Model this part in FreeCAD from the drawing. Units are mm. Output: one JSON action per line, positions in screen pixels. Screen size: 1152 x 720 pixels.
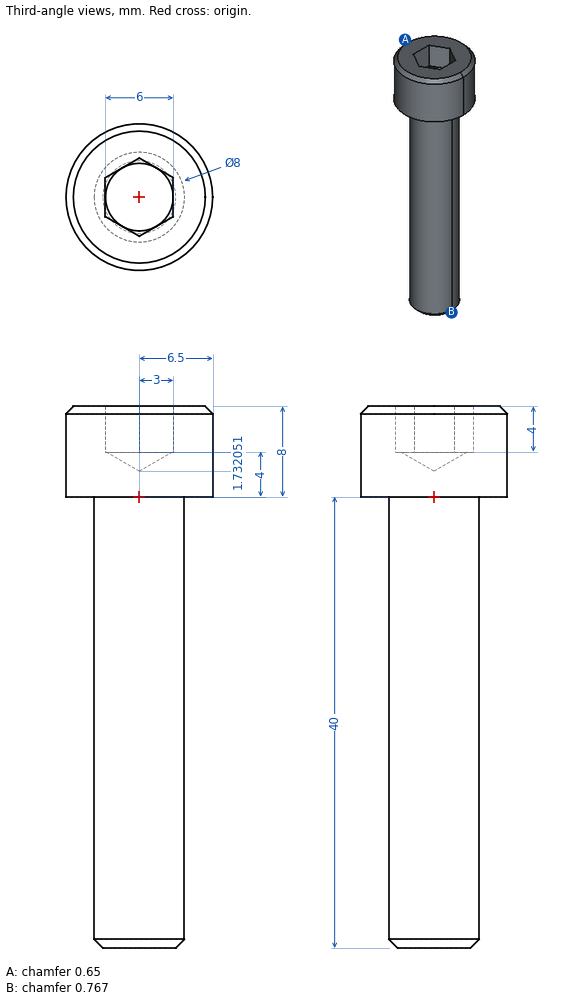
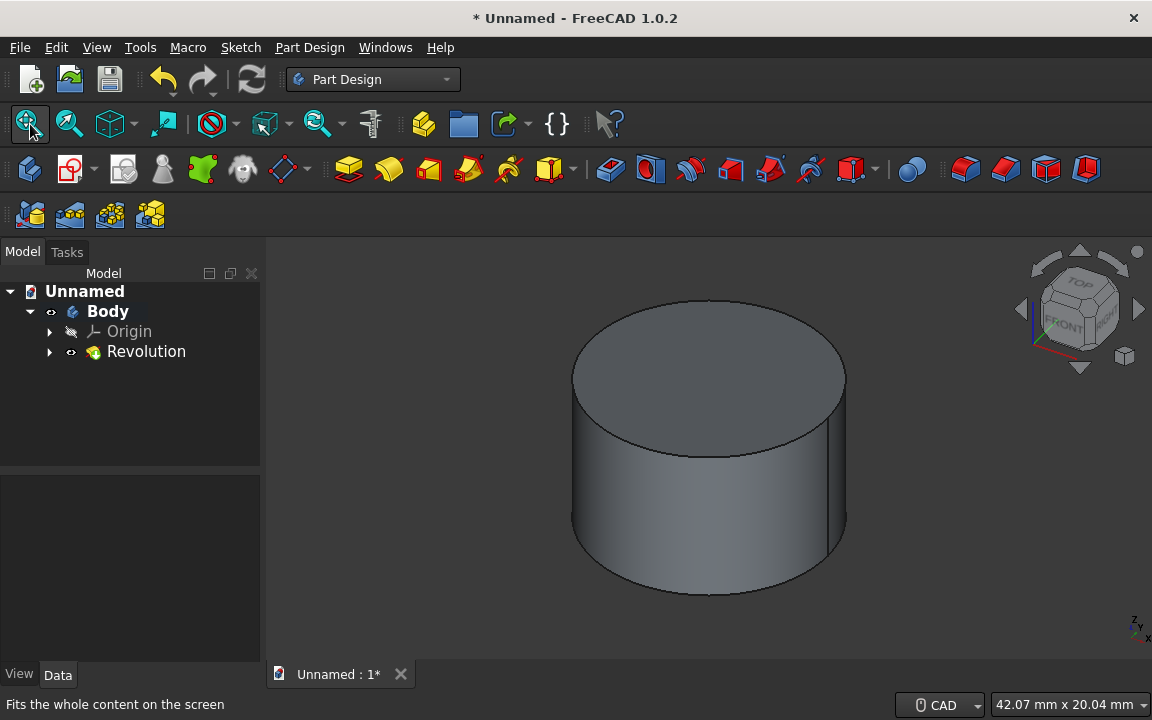
{"action": "key", "text": "5"}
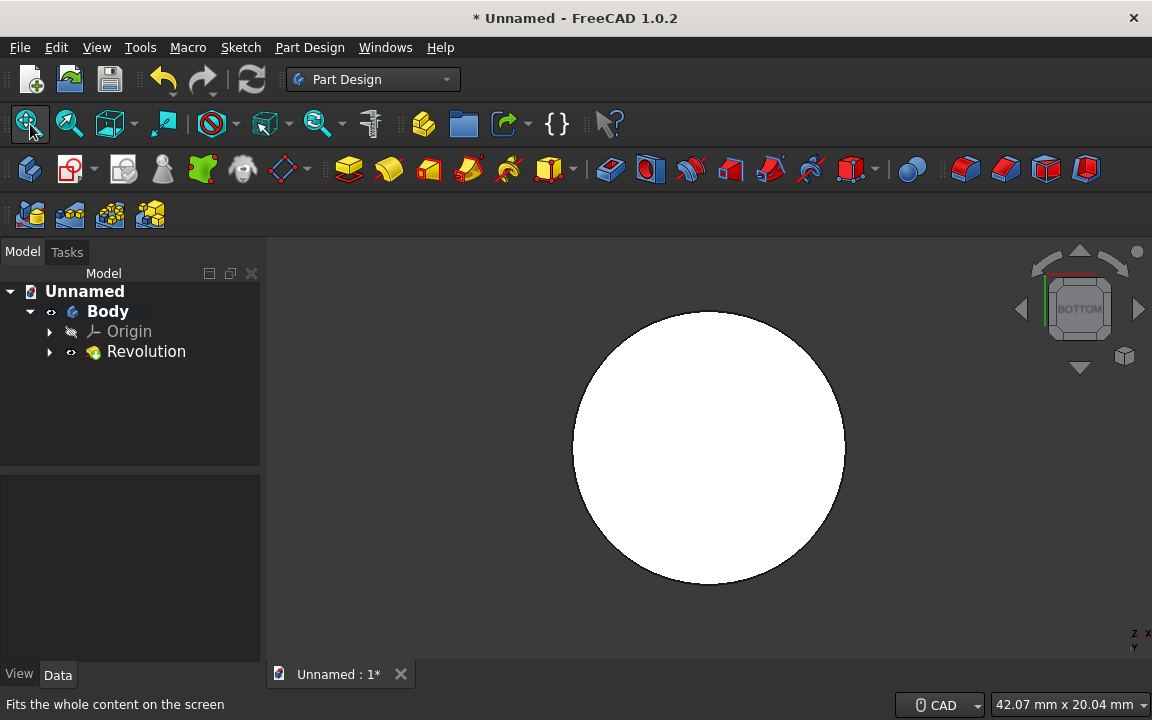
{"action": "left_click", "coordinate": [709, 447]}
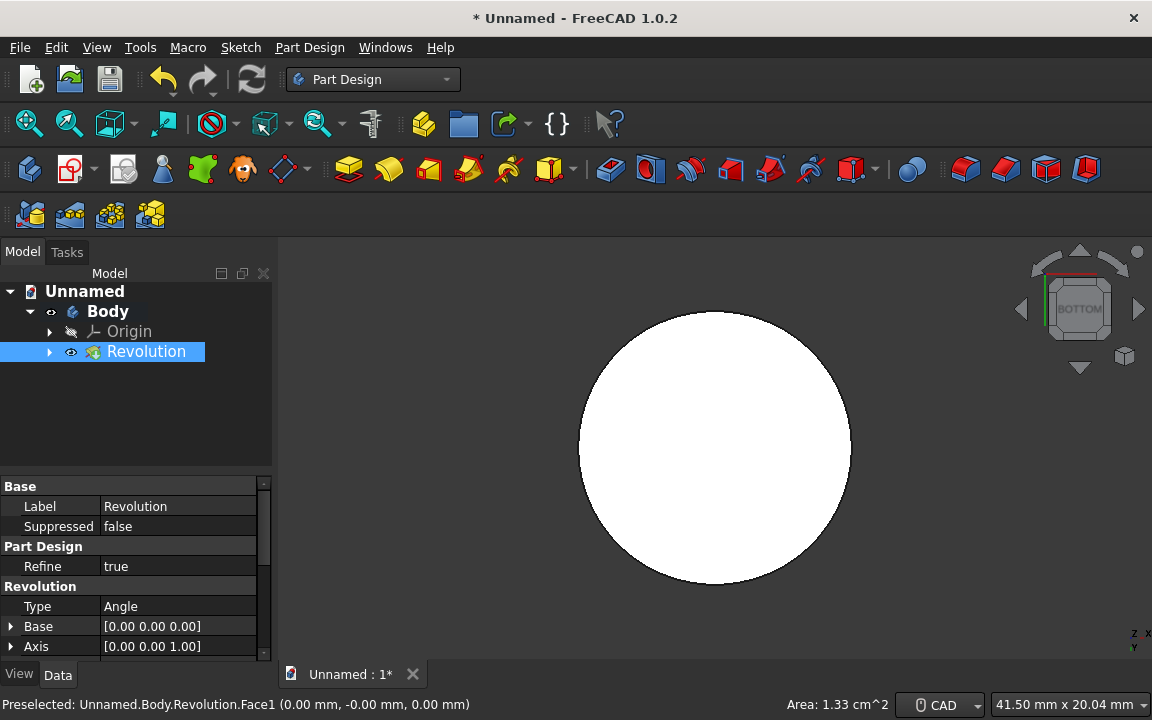
{"action": "left_click", "coordinate": [70, 170]}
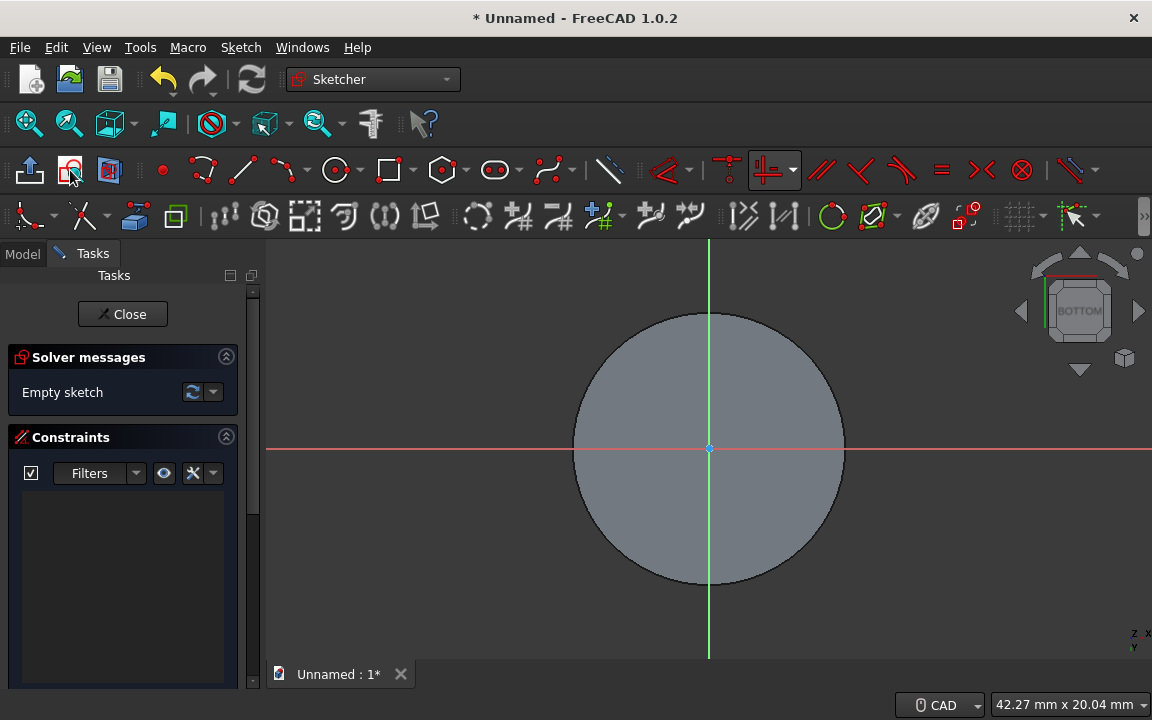
{"action": "scroll", "coordinate": [848, 449], "scroll_direction": "up", "scroll_amount": 2}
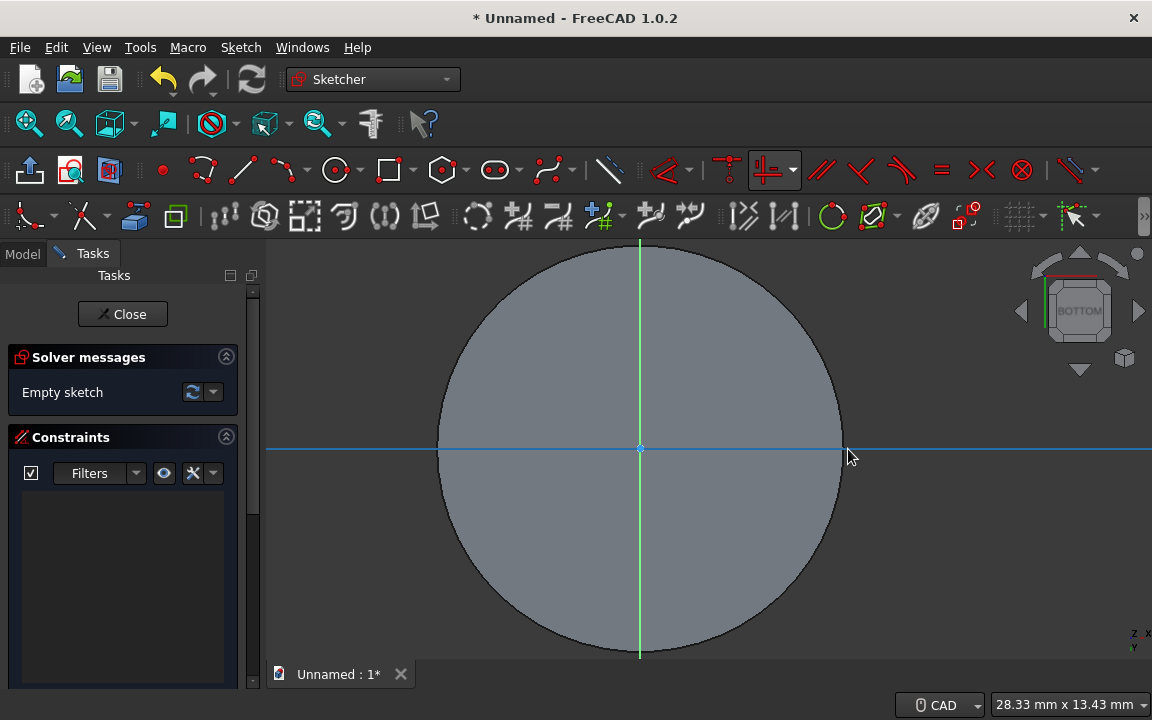
{"action": "left_click", "coordinate": [336, 170]}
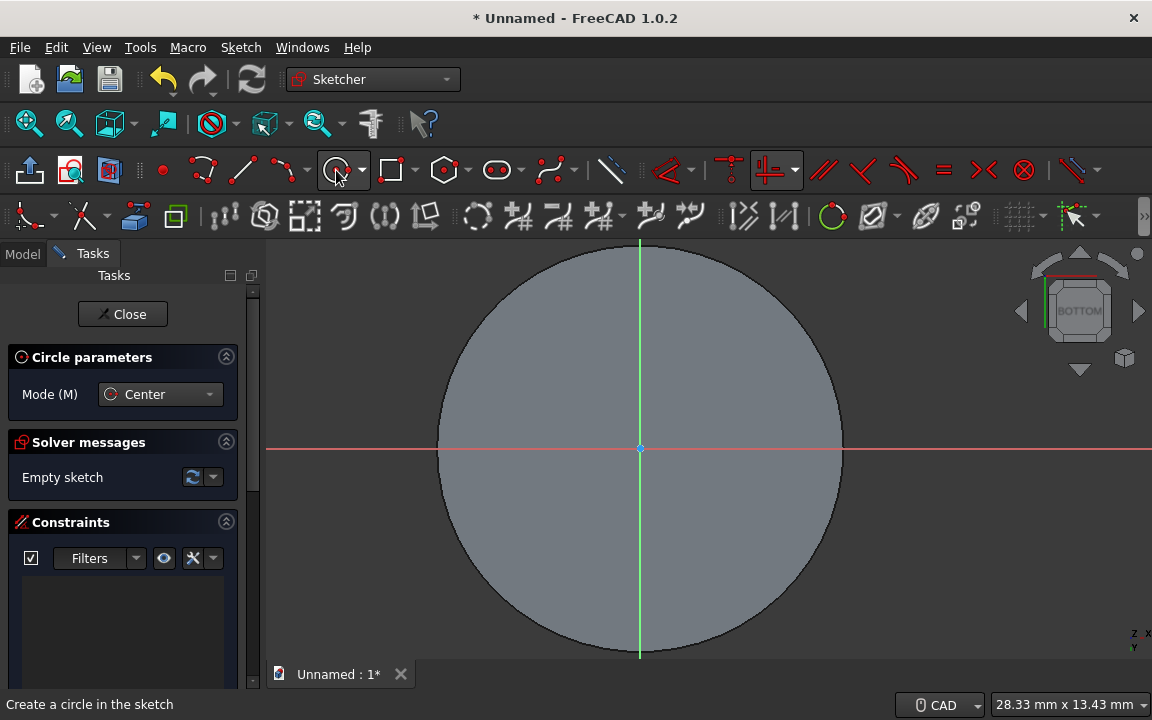
{"action": "left_click", "coordinate": [640, 449]}
{"action": "mouse_move", "coordinate": [729, 360]}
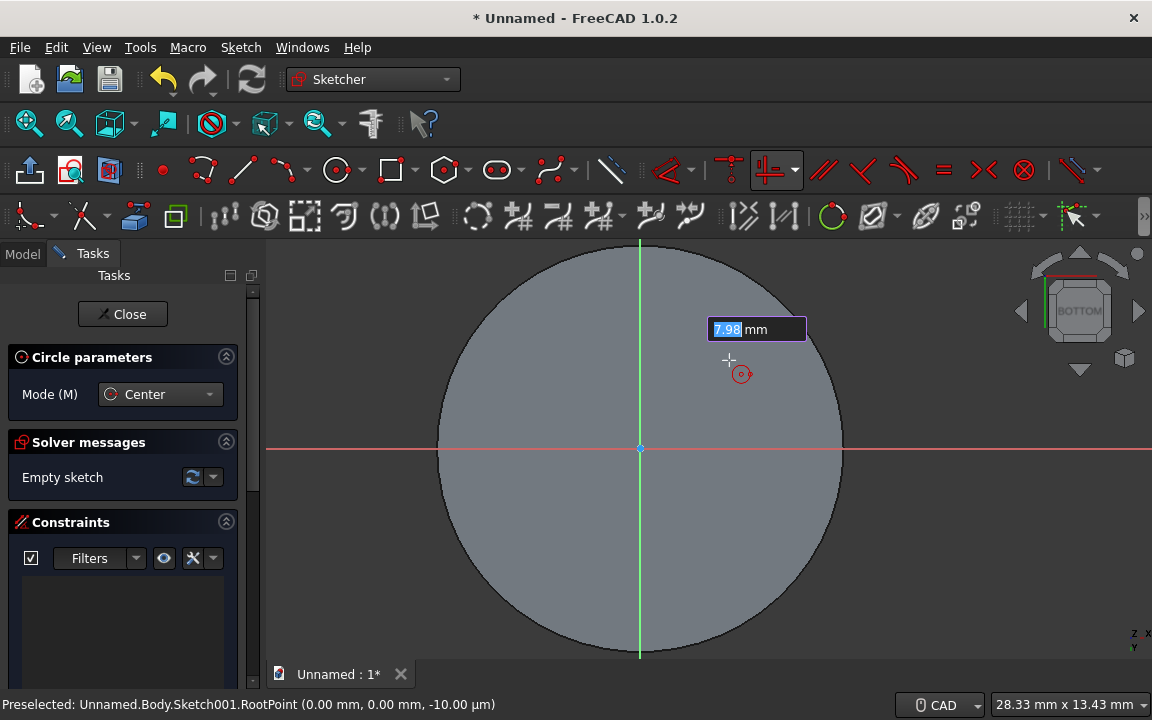
{"action": "type", "text": "8"}
{"action": "key", "text": "Return"}
{"action": "key", "text": "Escape"}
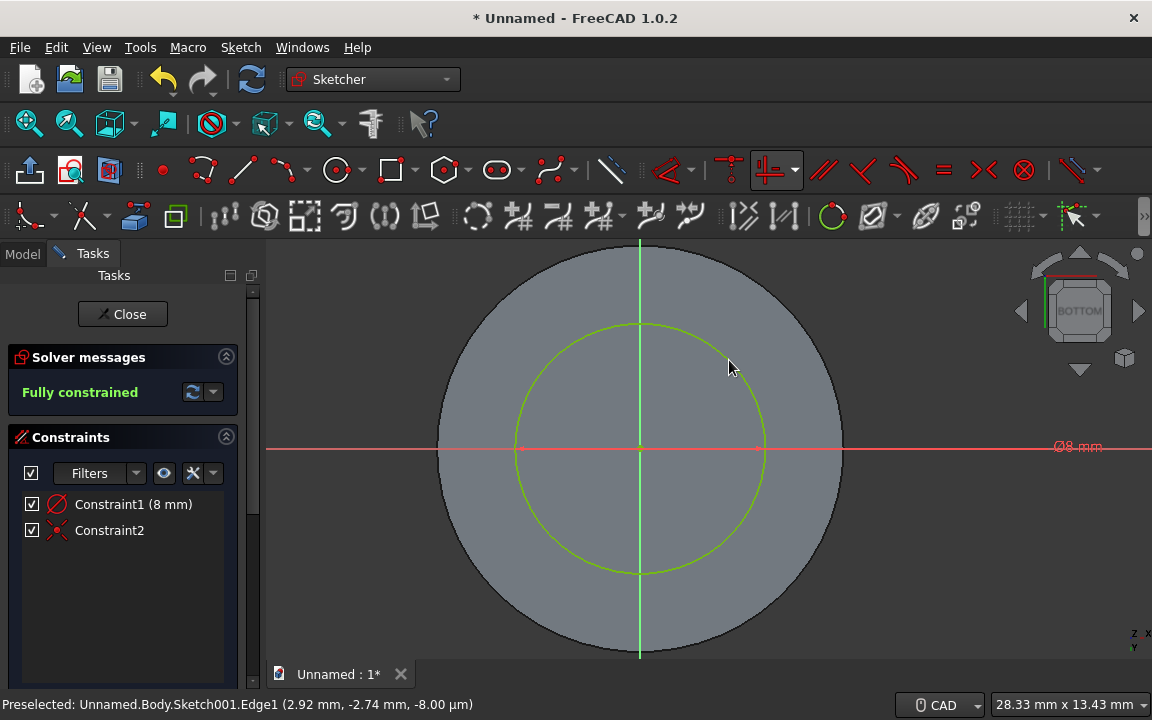
{"action": "left_click", "coordinate": [123, 314]}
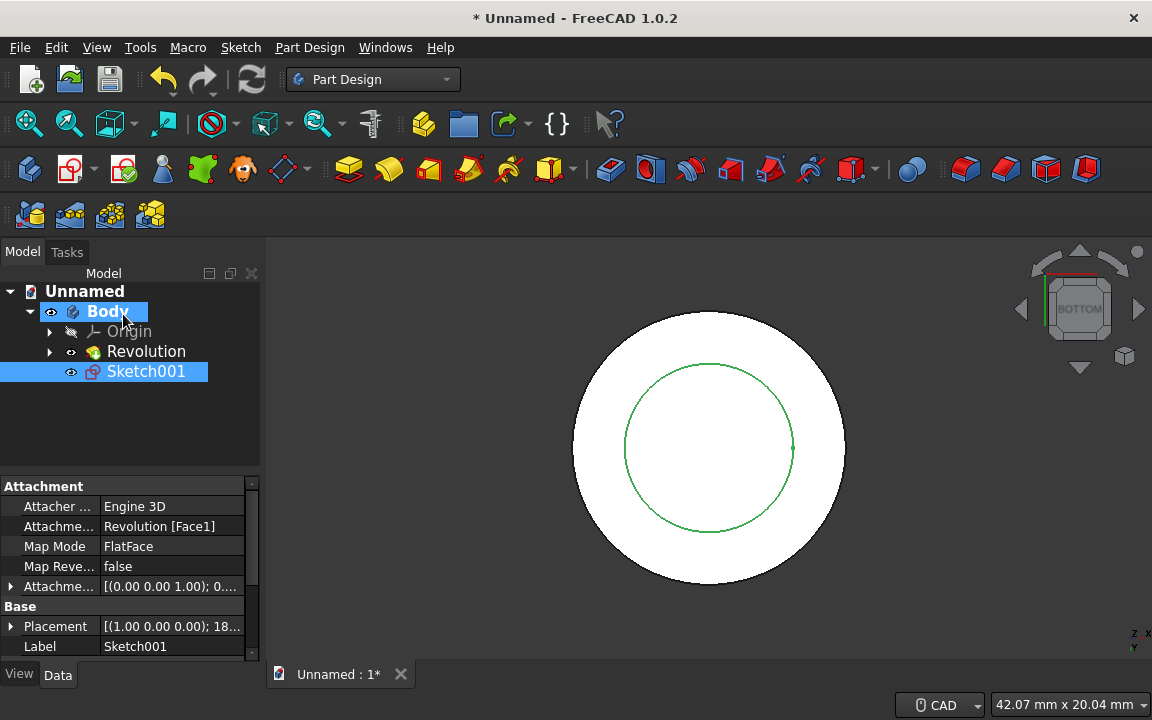
{"action": "left_click", "coordinate": [350, 170]}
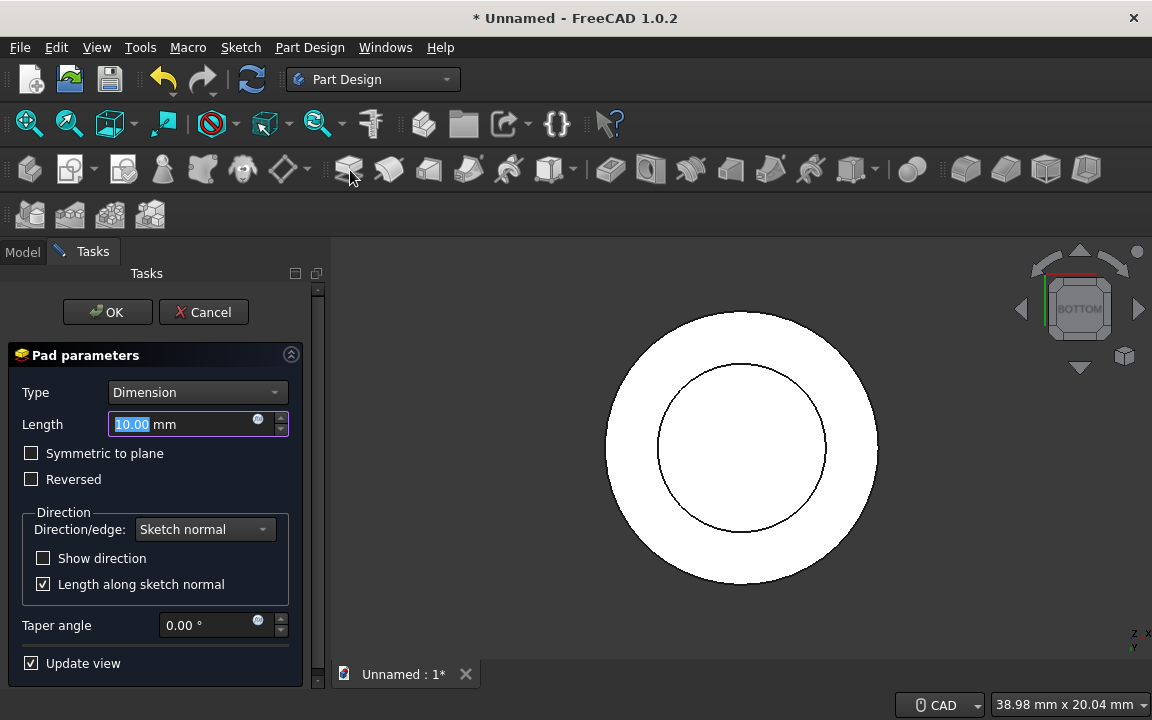
{"action": "type", "text": "40"}
{"action": "key", "text": "Tab"}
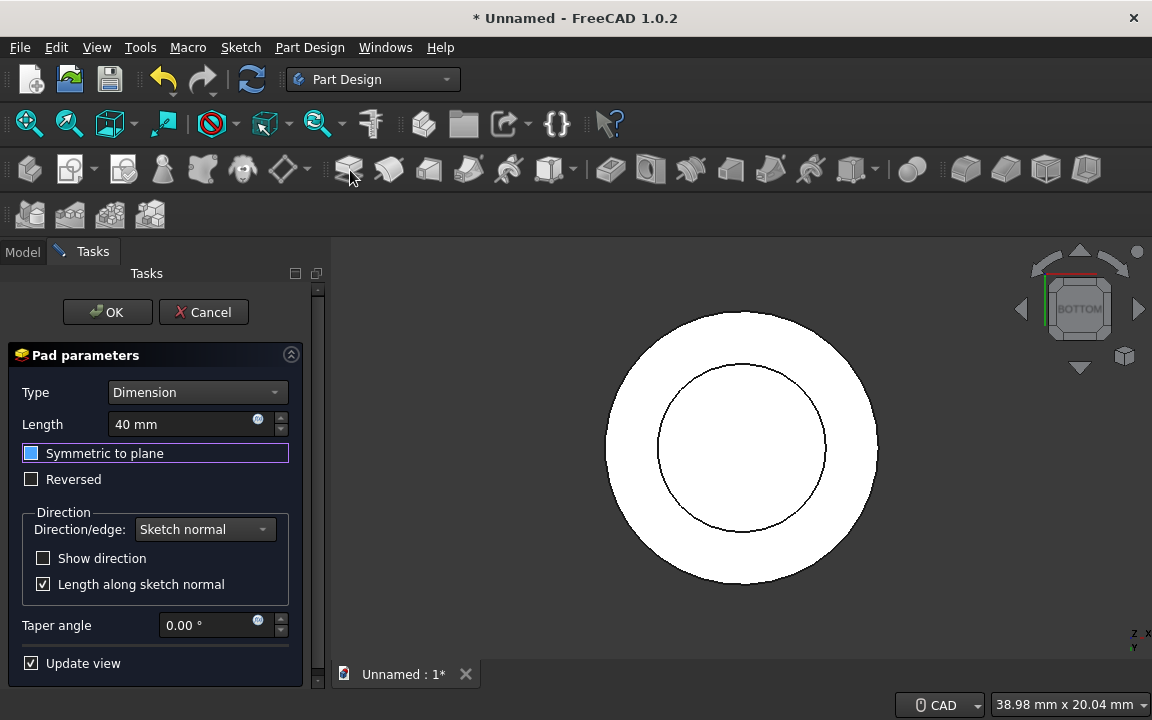
{"action": "left_click", "coordinate": [108, 312]}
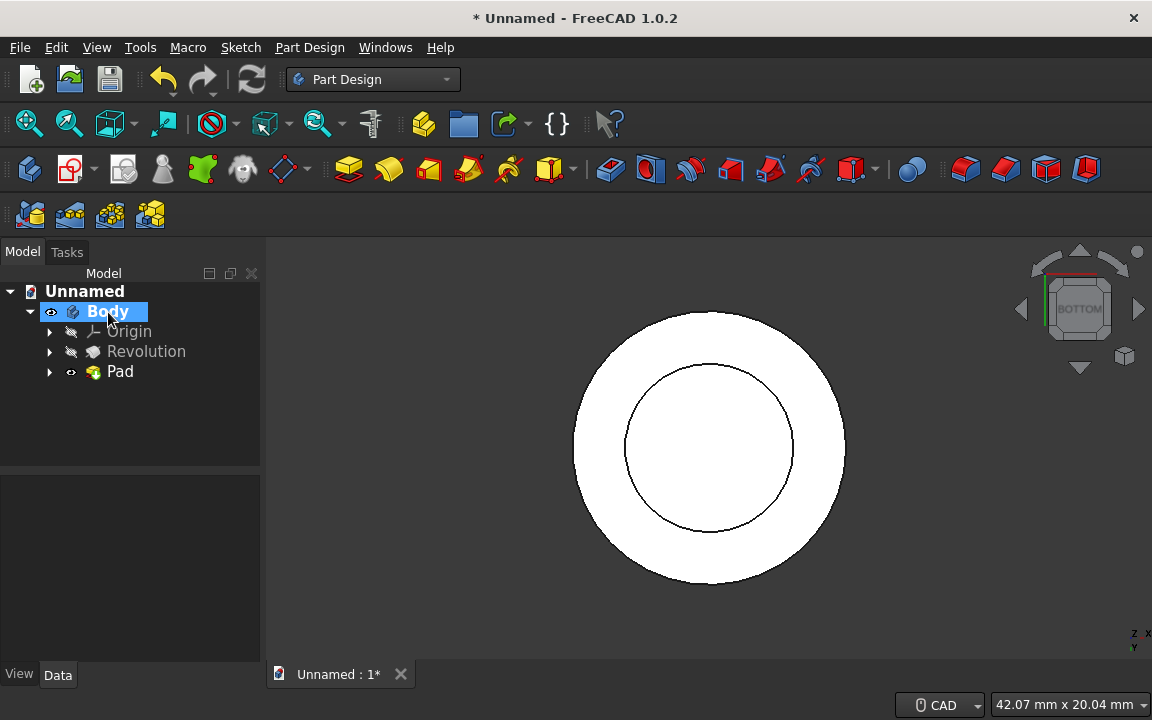
{"action": "key", "text": "0"}